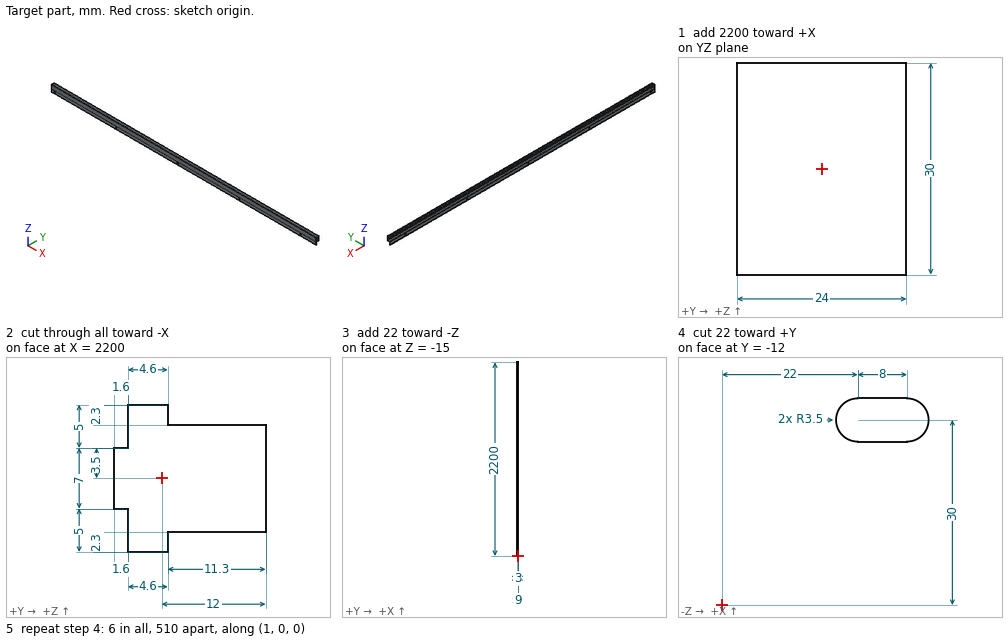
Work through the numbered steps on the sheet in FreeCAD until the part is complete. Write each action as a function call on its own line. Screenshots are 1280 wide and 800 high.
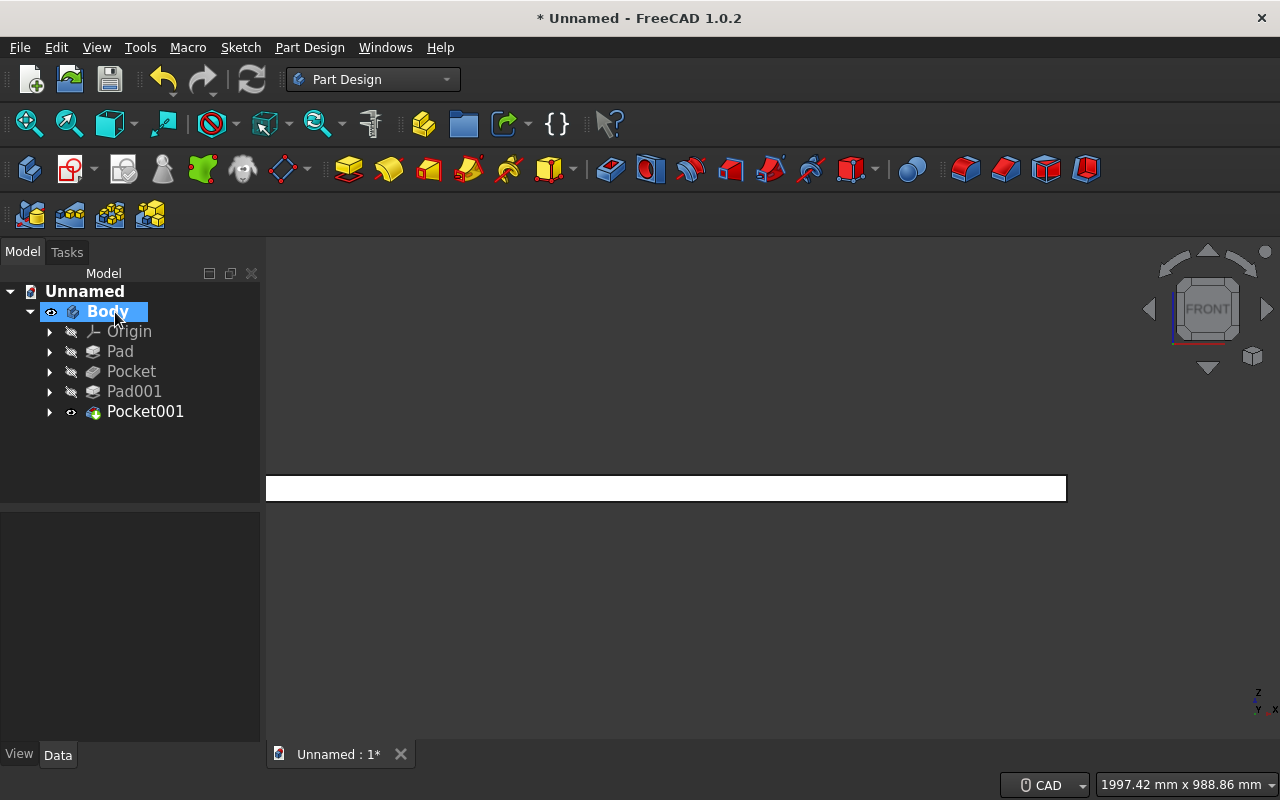
click(30, 124)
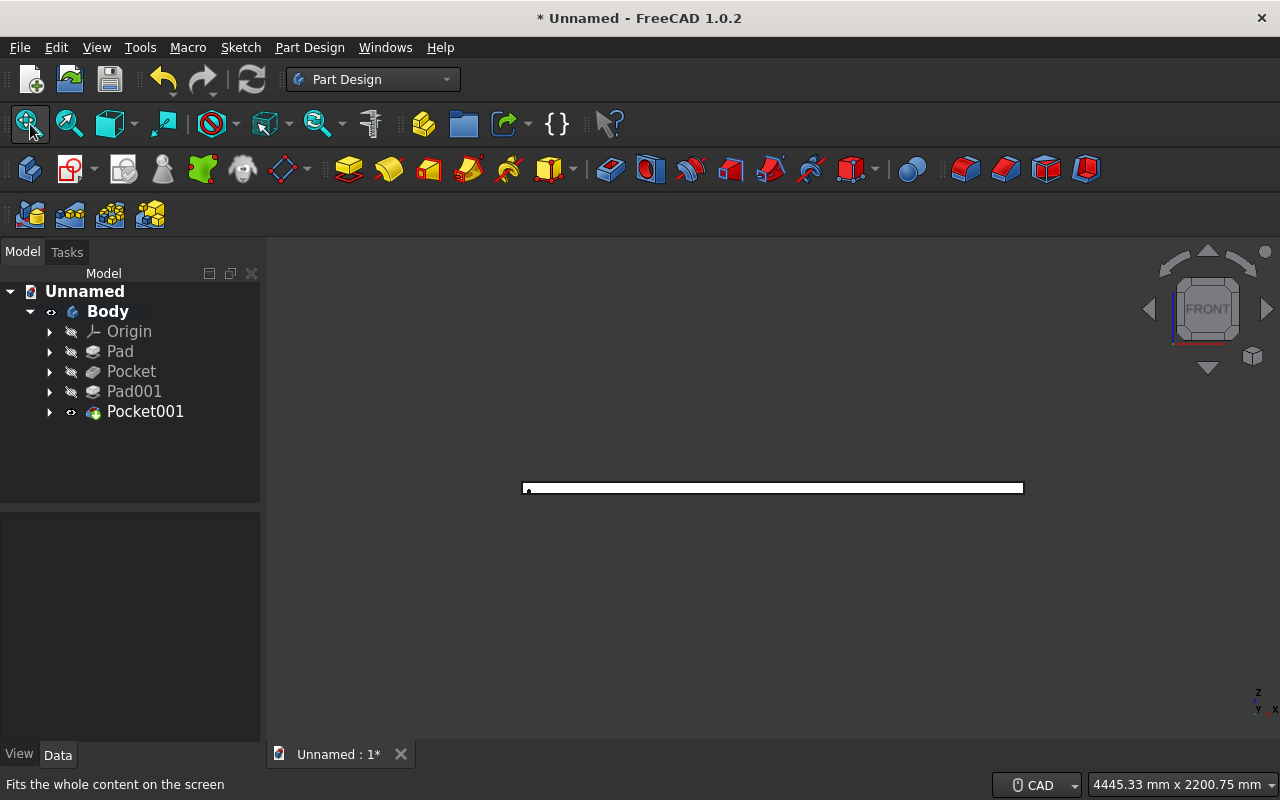
click(116, 412)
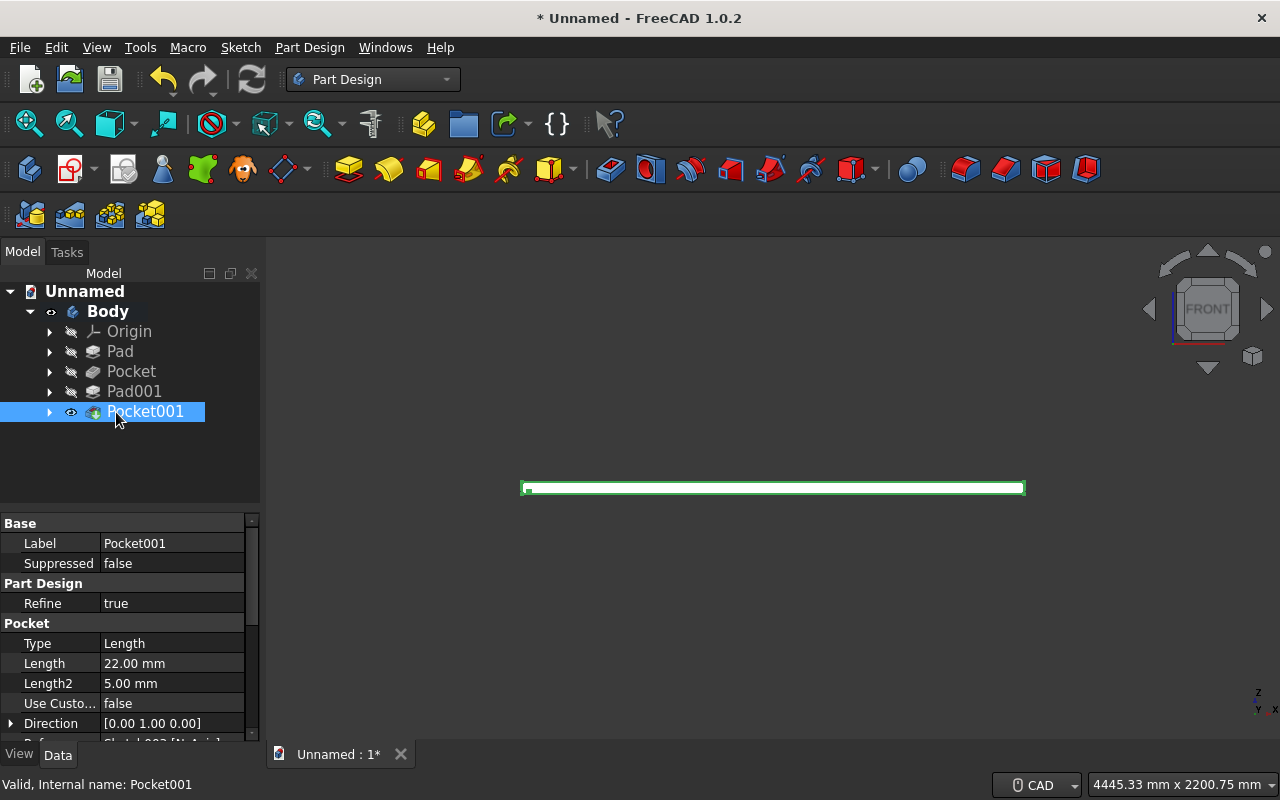
click(70, 214)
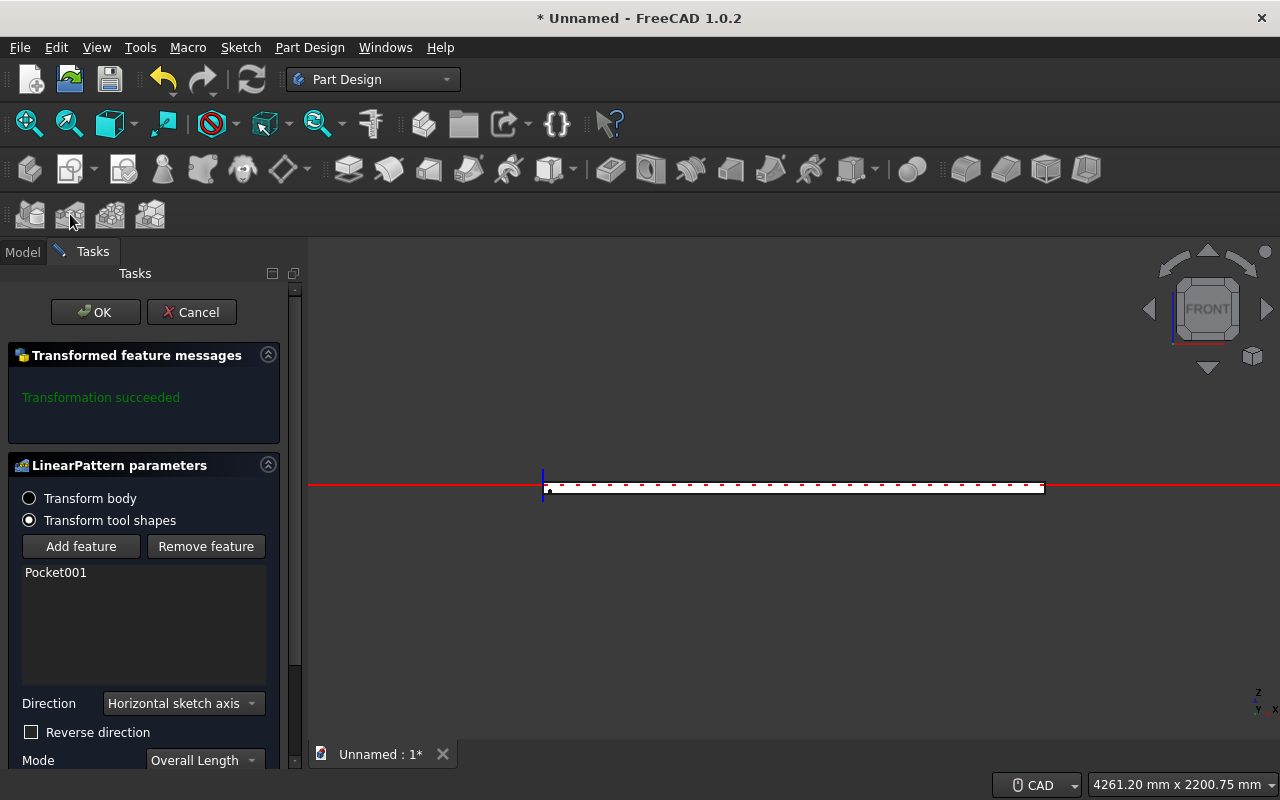
click(184, 704)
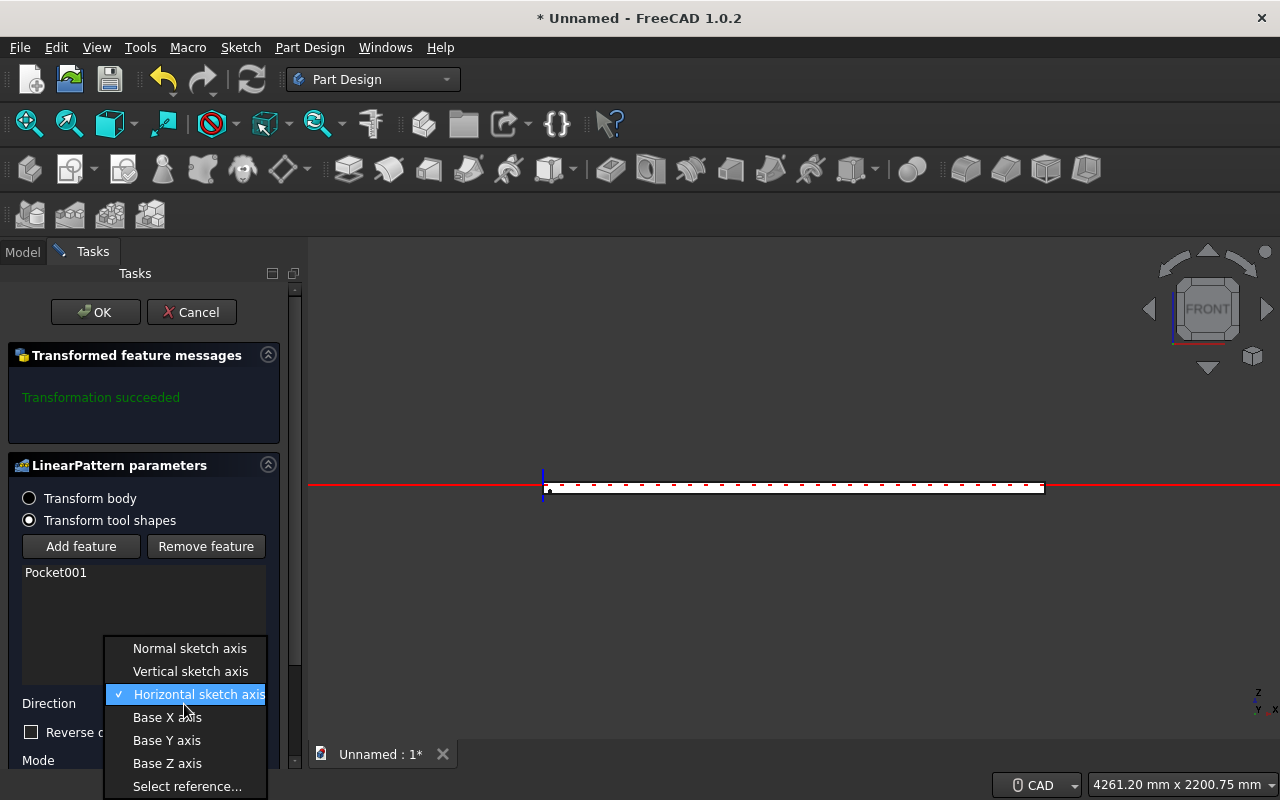
click(184, 718)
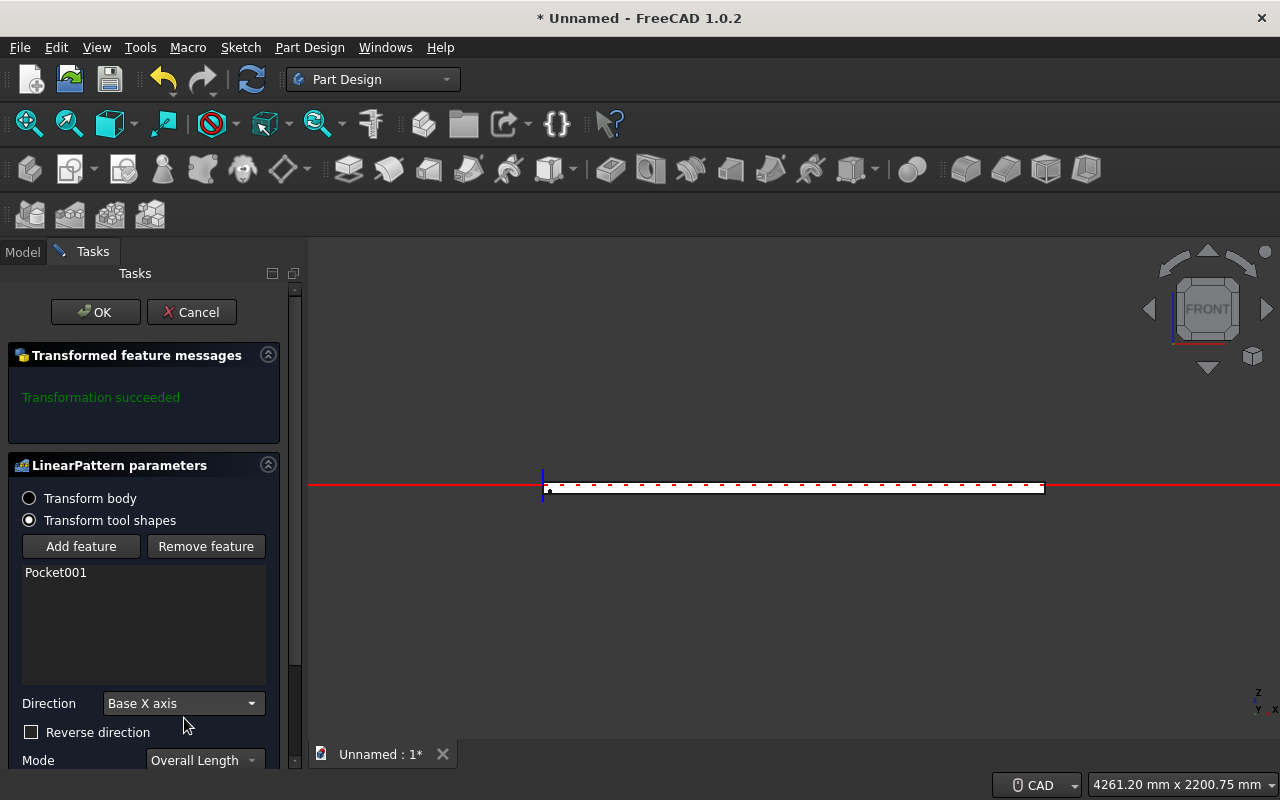
scroll(295, 526, down, 2)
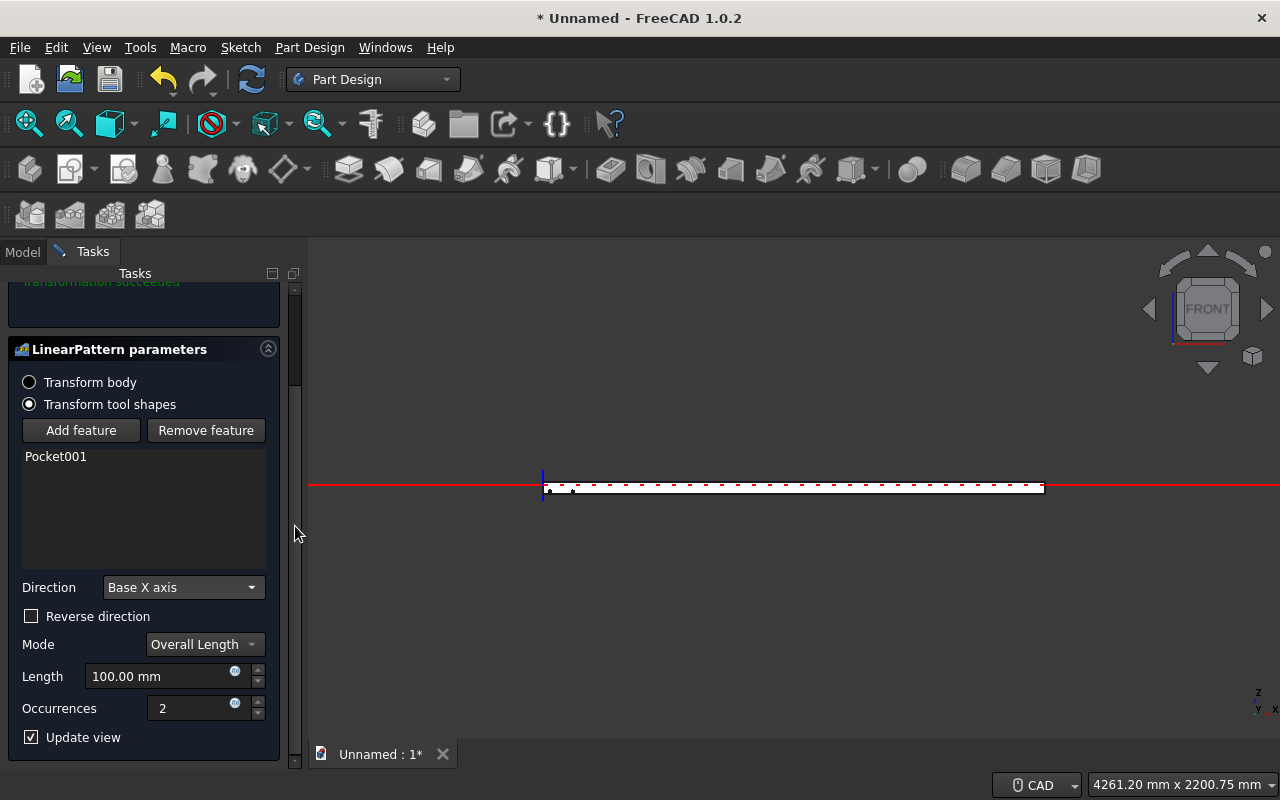
click(206, 644)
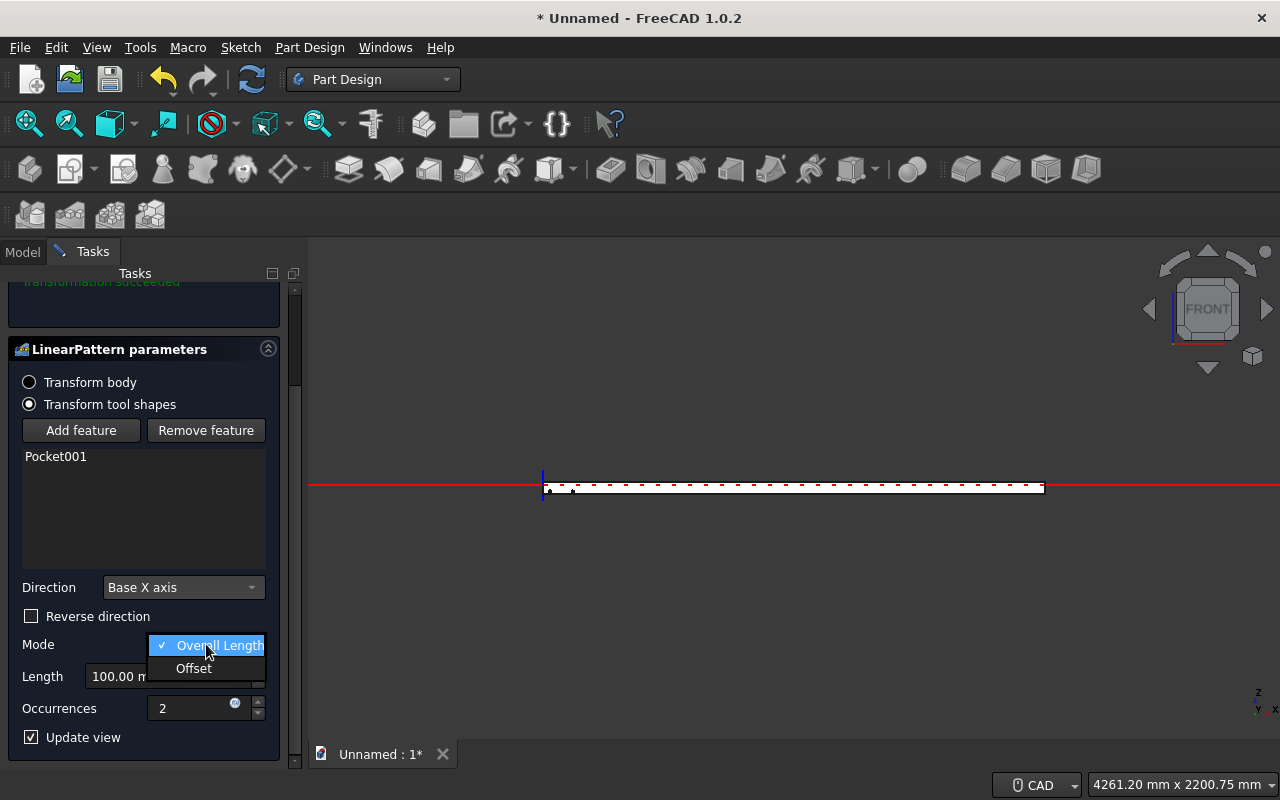
click(206, 668)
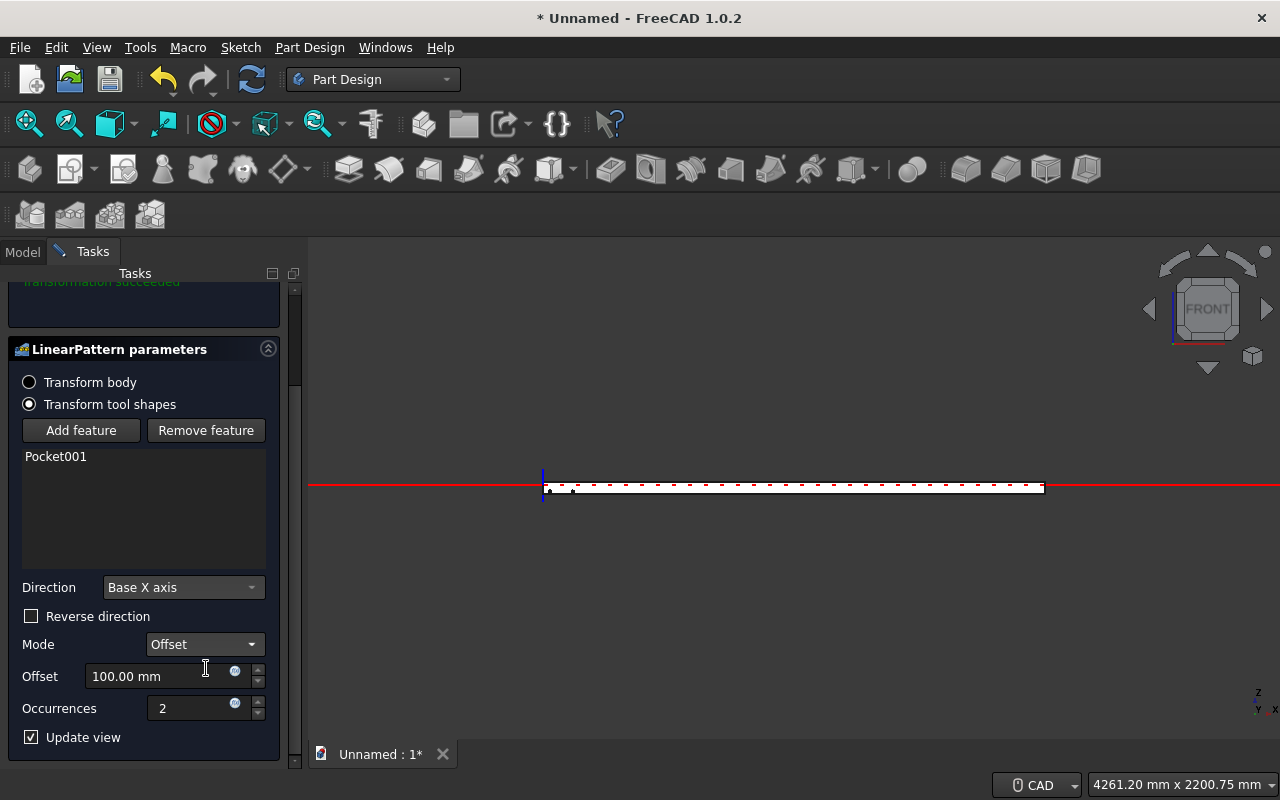
triple_click(168, 676)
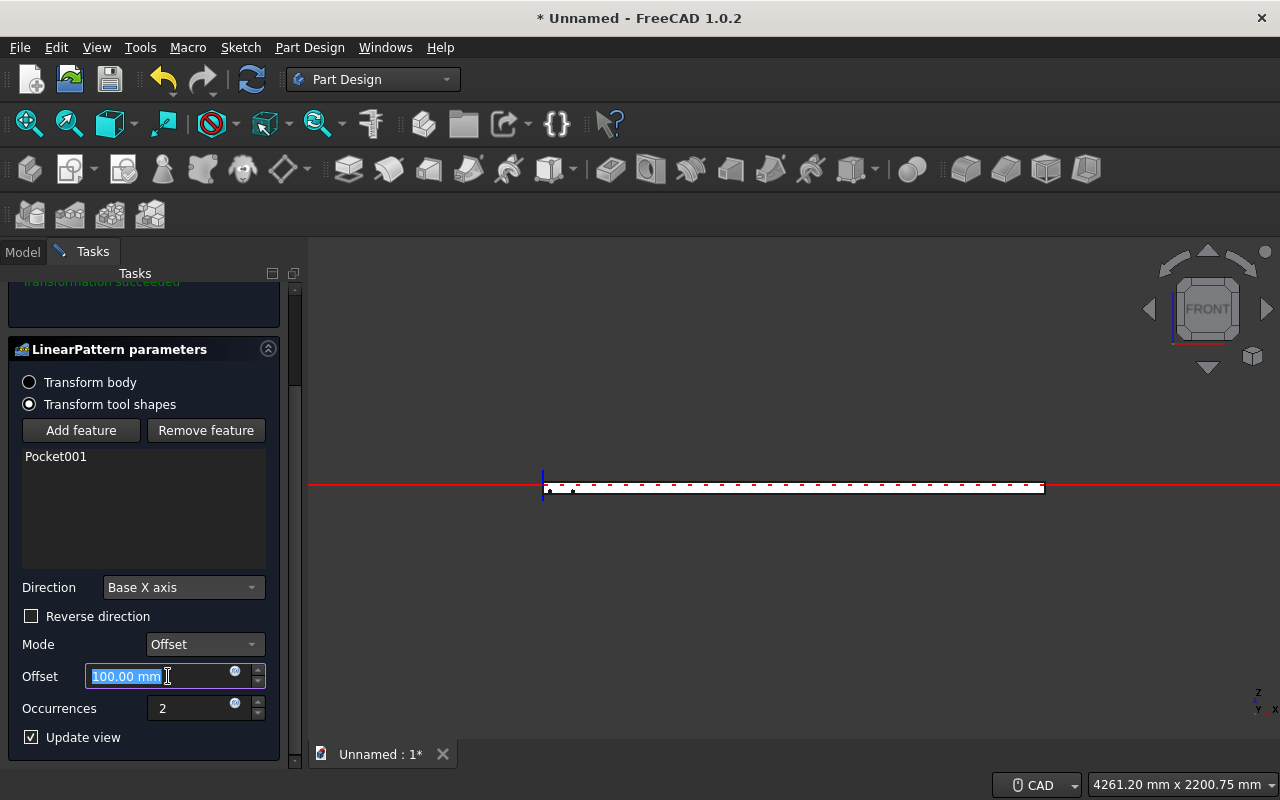
text(510)
key(Tab)